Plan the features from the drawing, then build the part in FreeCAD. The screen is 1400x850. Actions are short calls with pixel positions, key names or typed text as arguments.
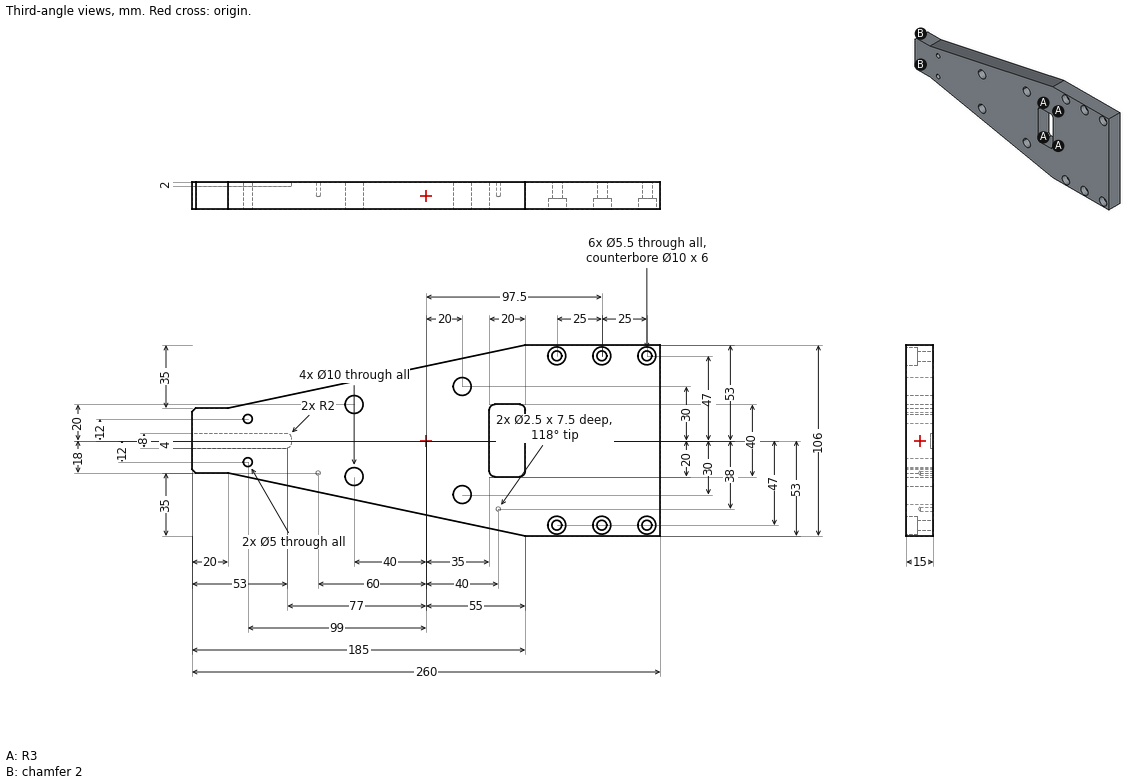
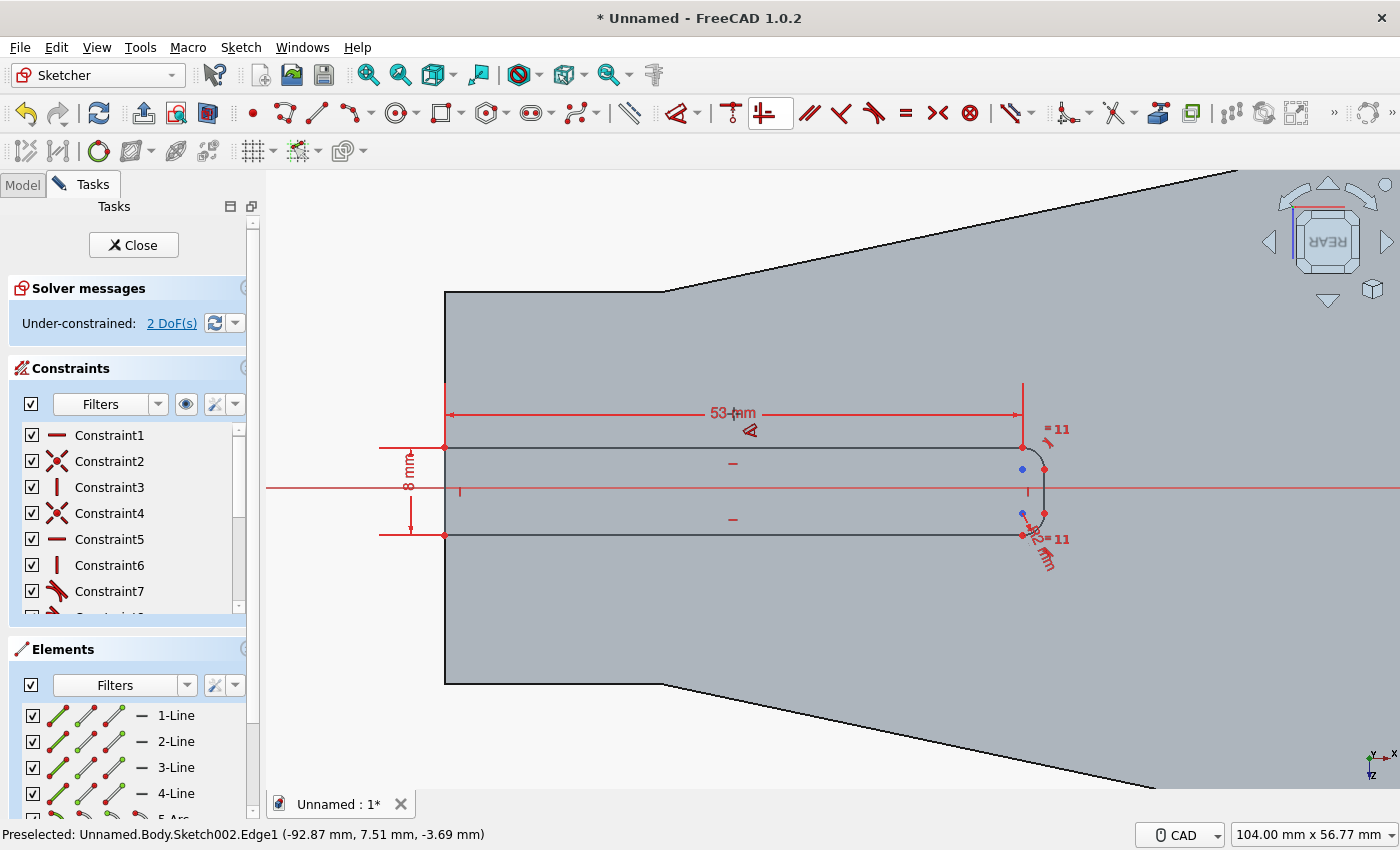
click(1023, 448)
click(989, 468)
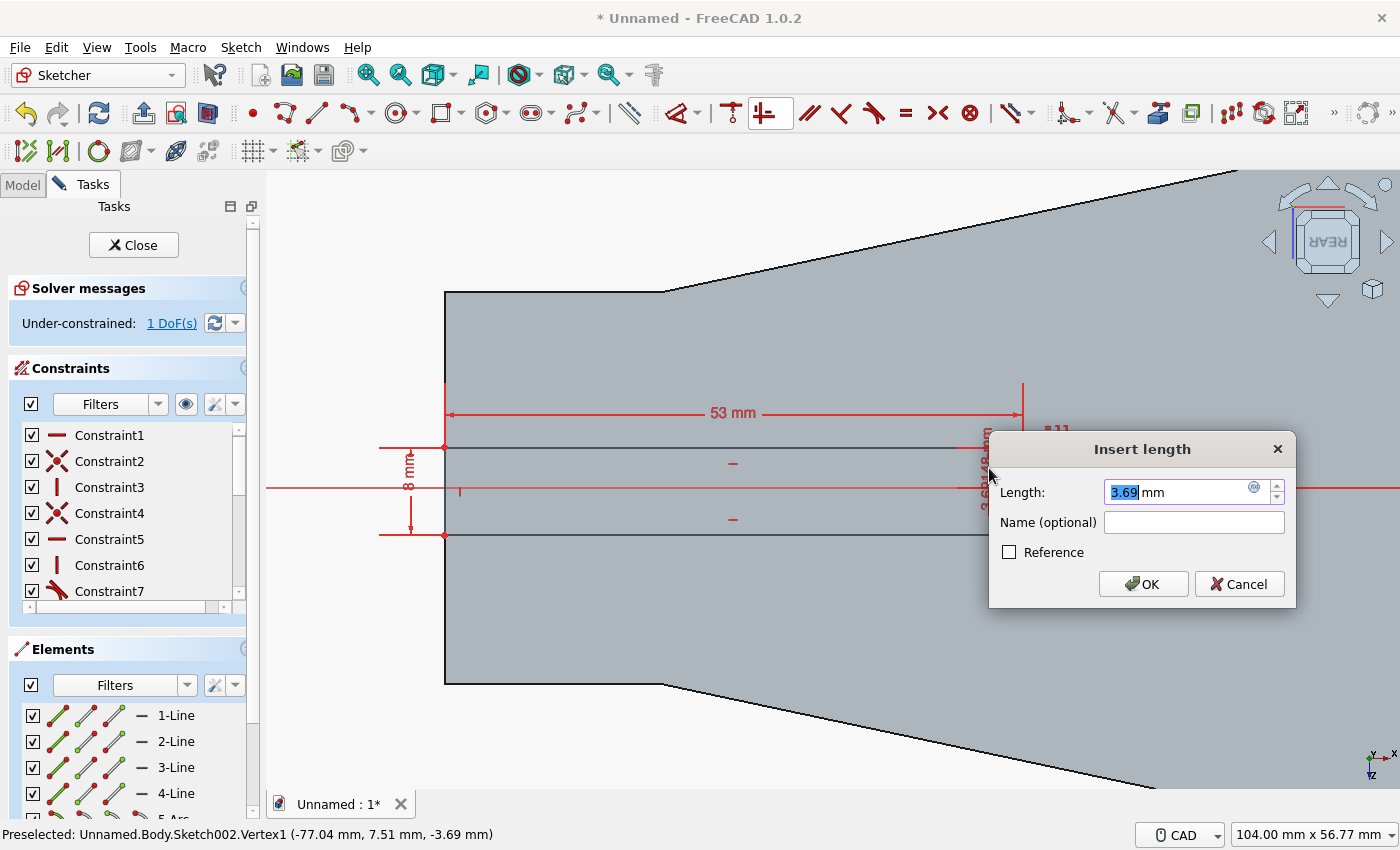
text(4)
key(Return)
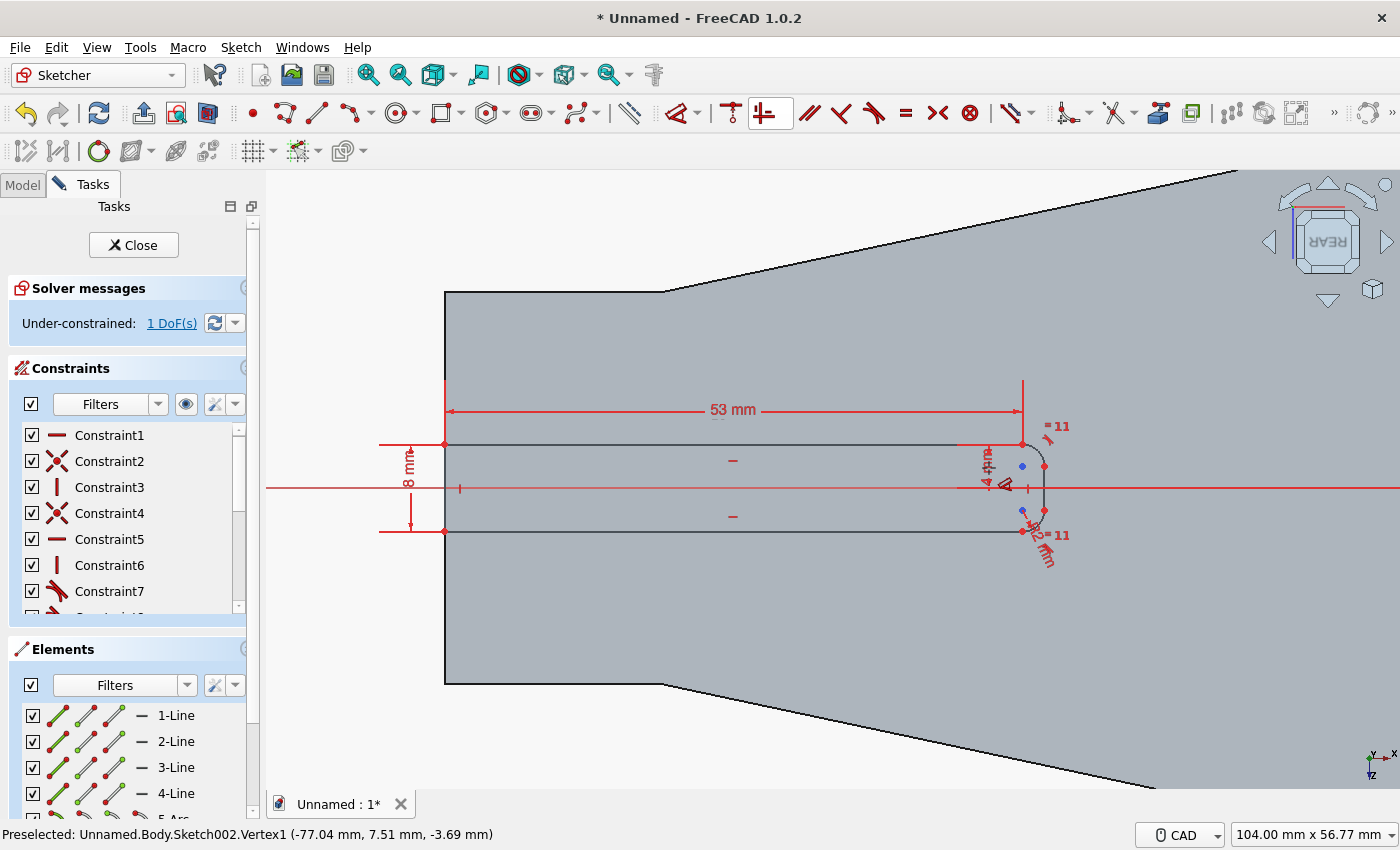
click(1023, 445)
click(1129, 411)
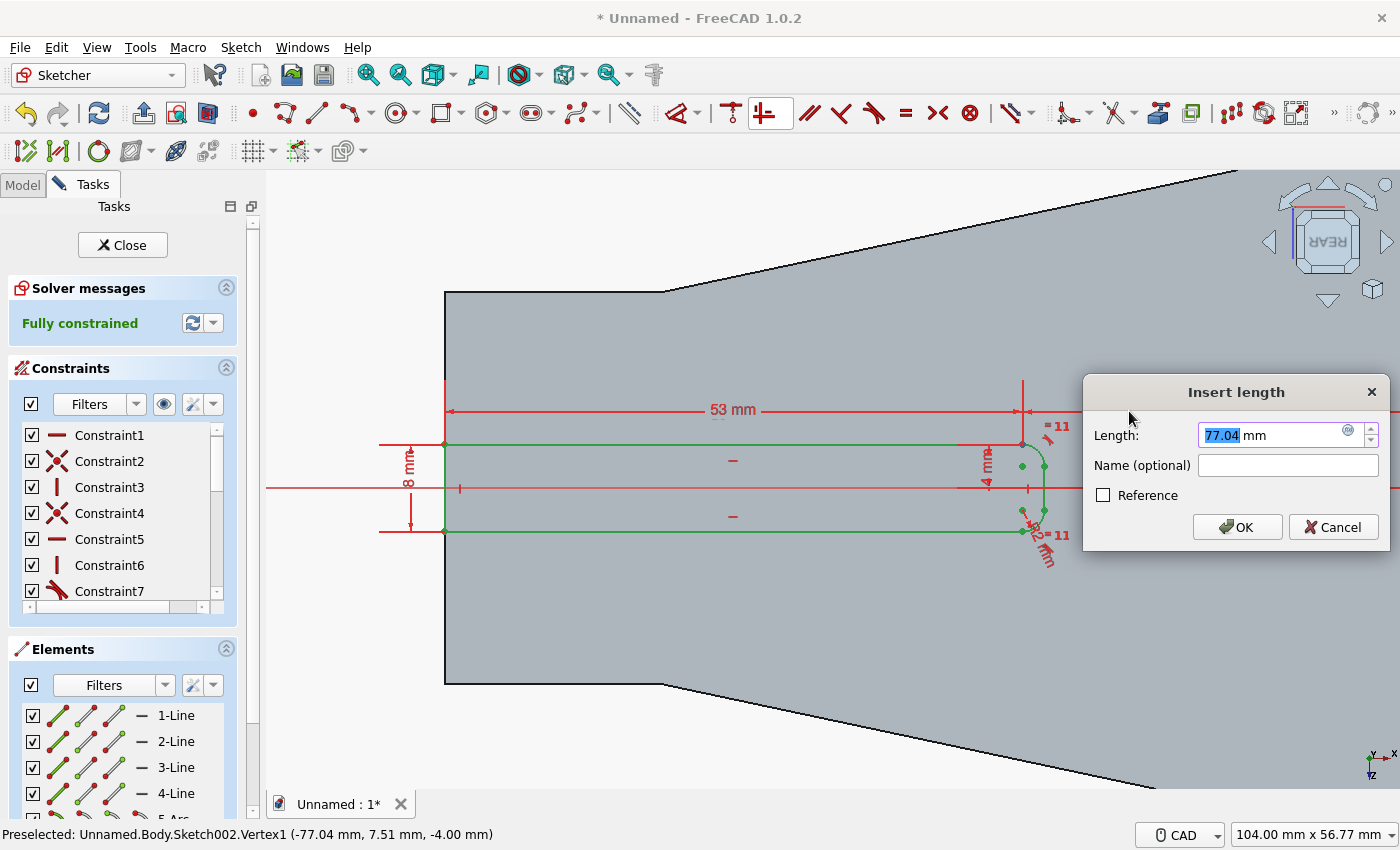
text(77)
key(Return)
key(Escape)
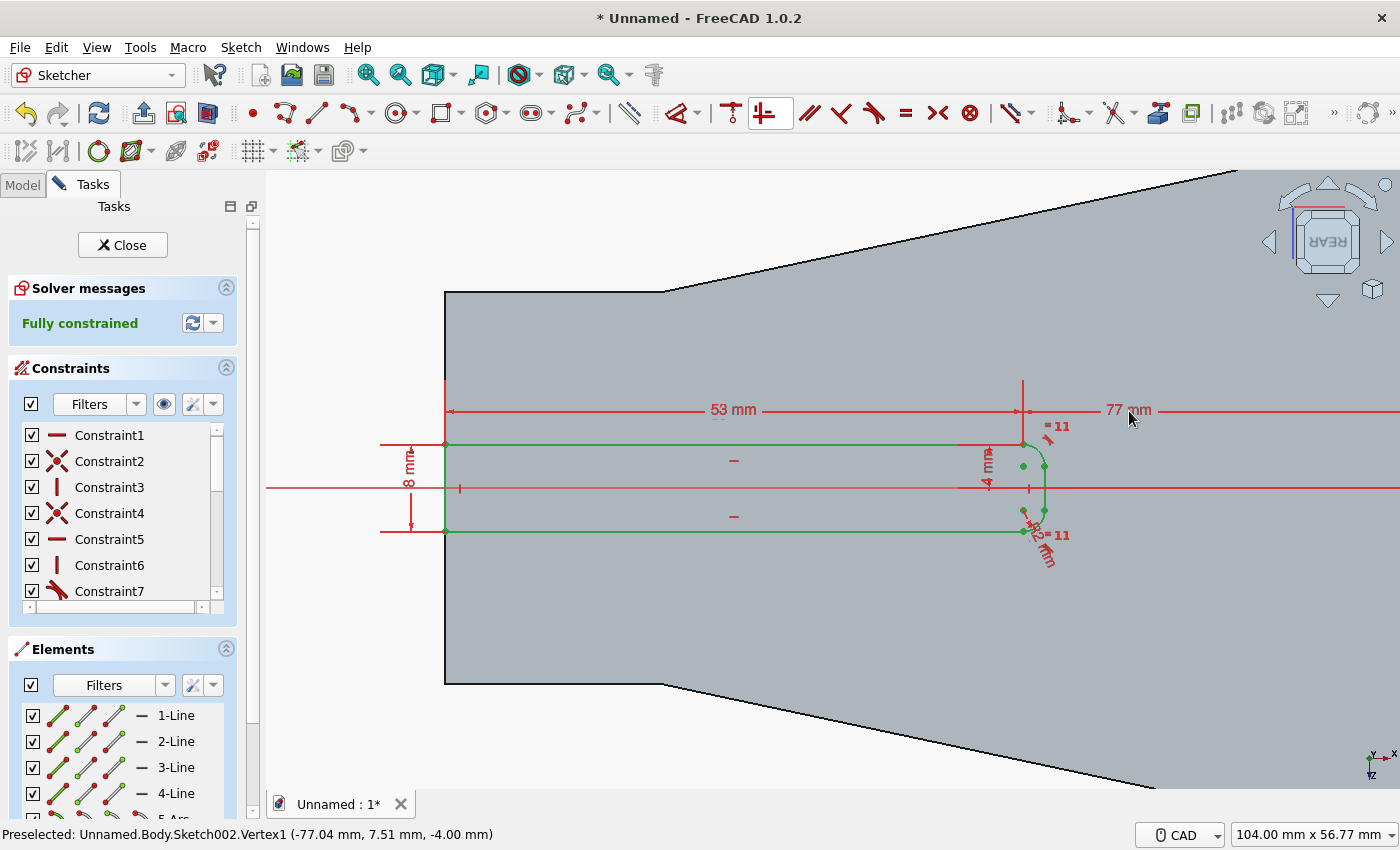
click(123, 245)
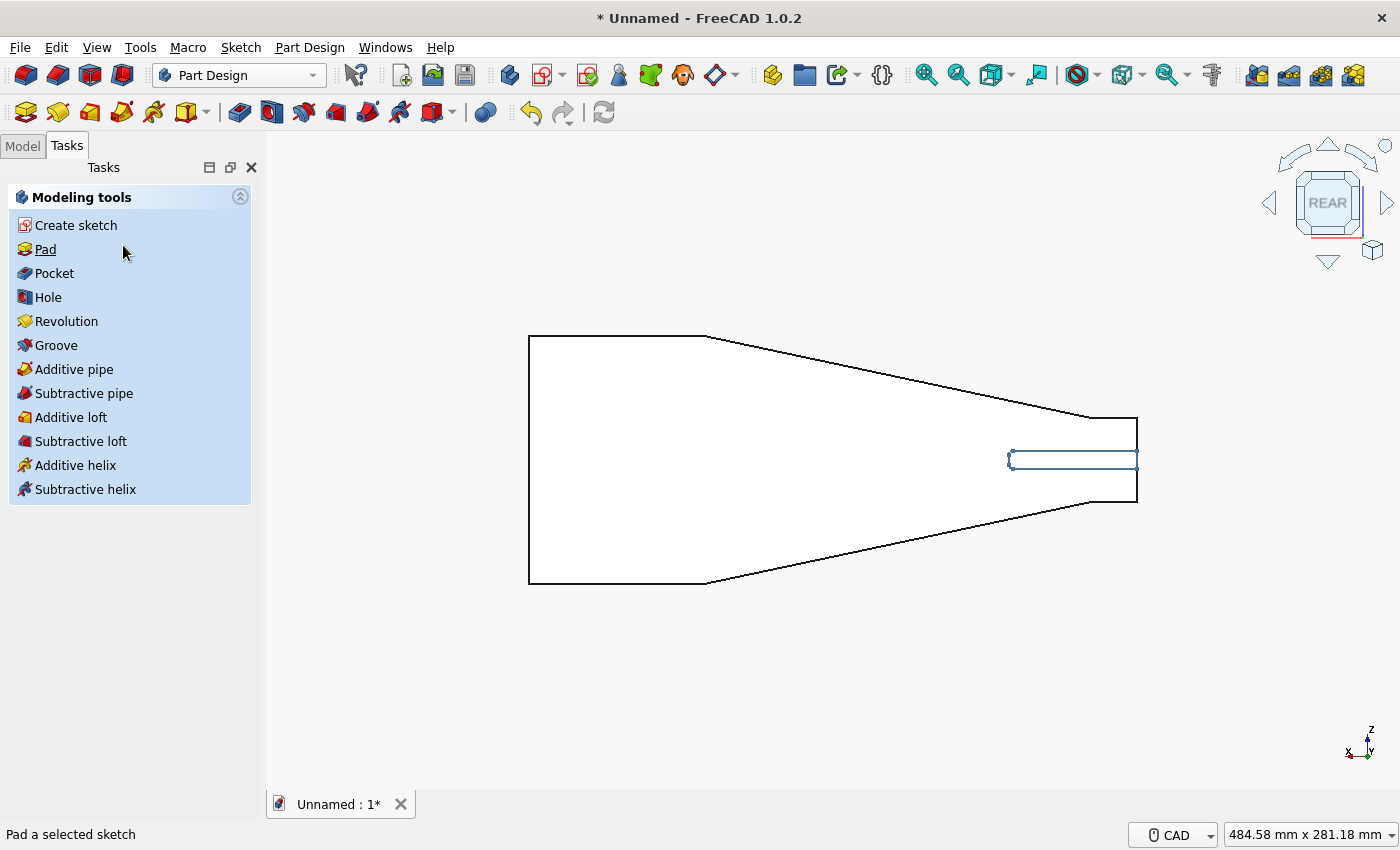
click(240, 112)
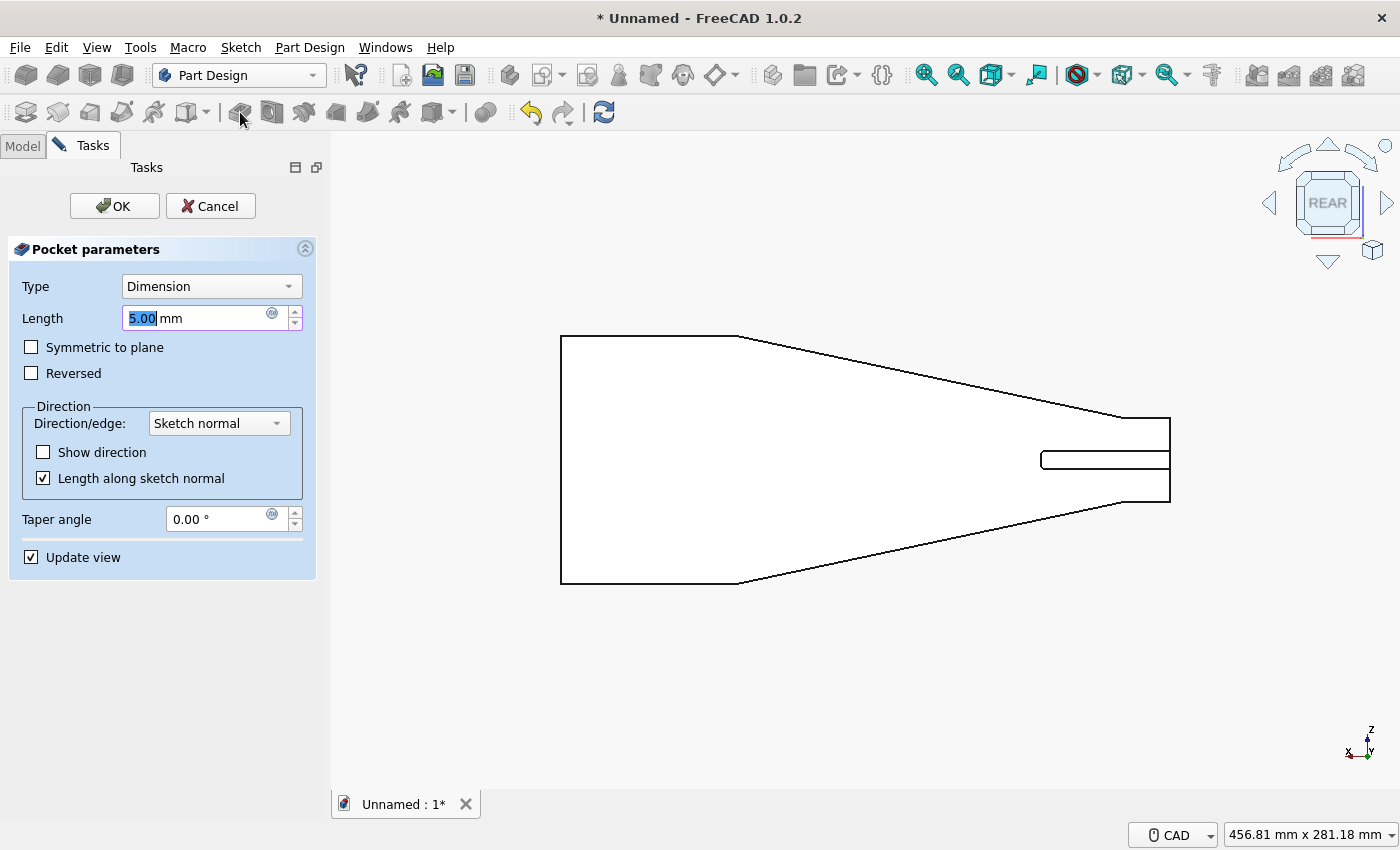
text(2)
key(Tab)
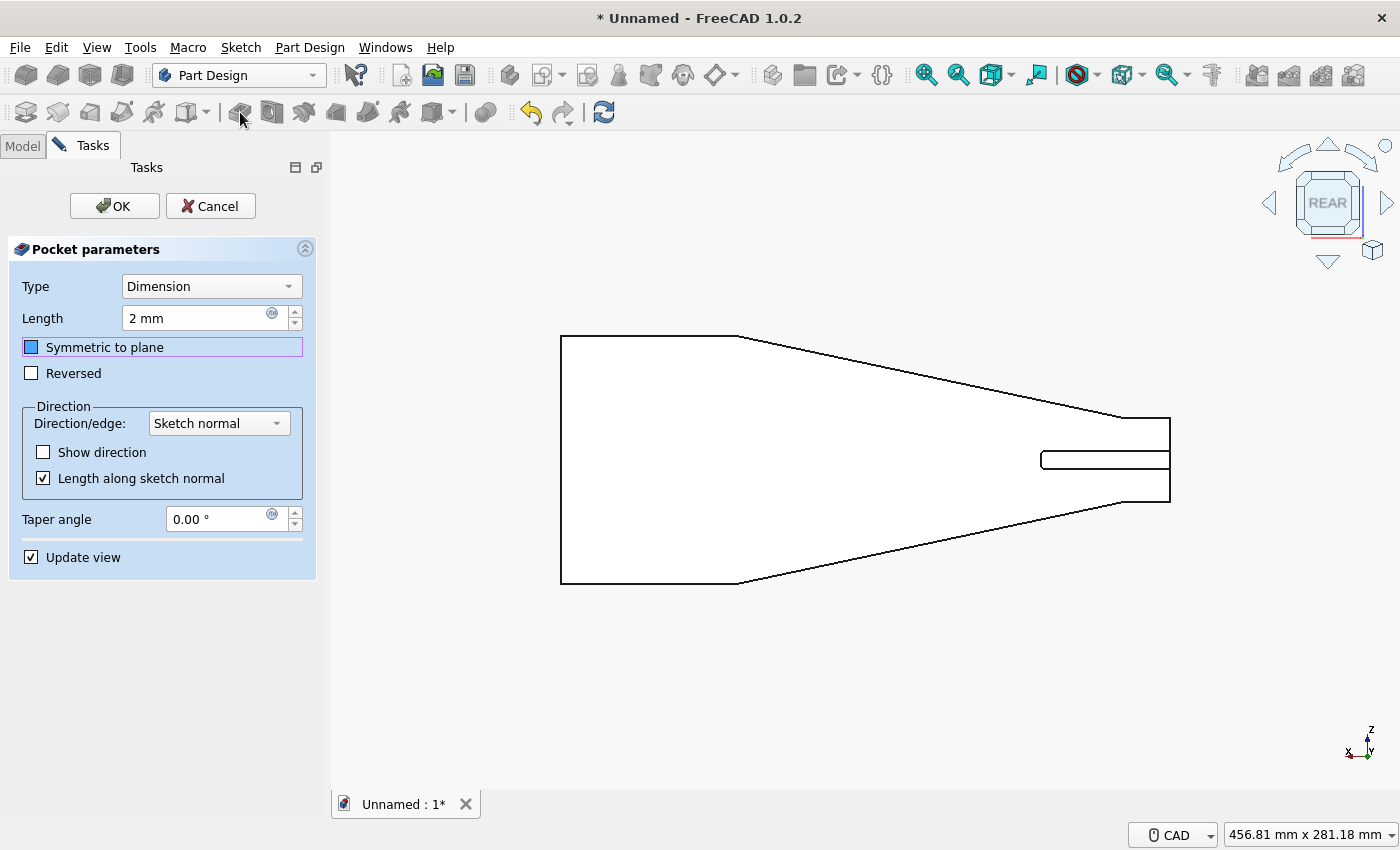
click(115, 206)